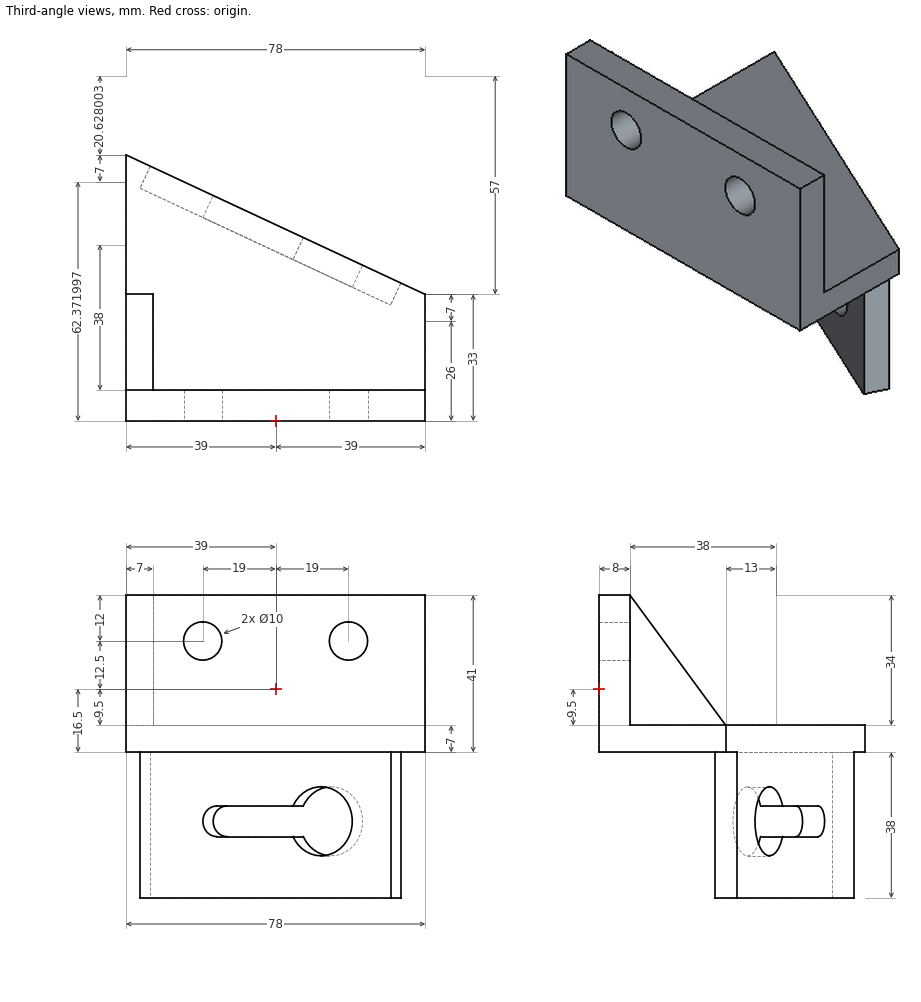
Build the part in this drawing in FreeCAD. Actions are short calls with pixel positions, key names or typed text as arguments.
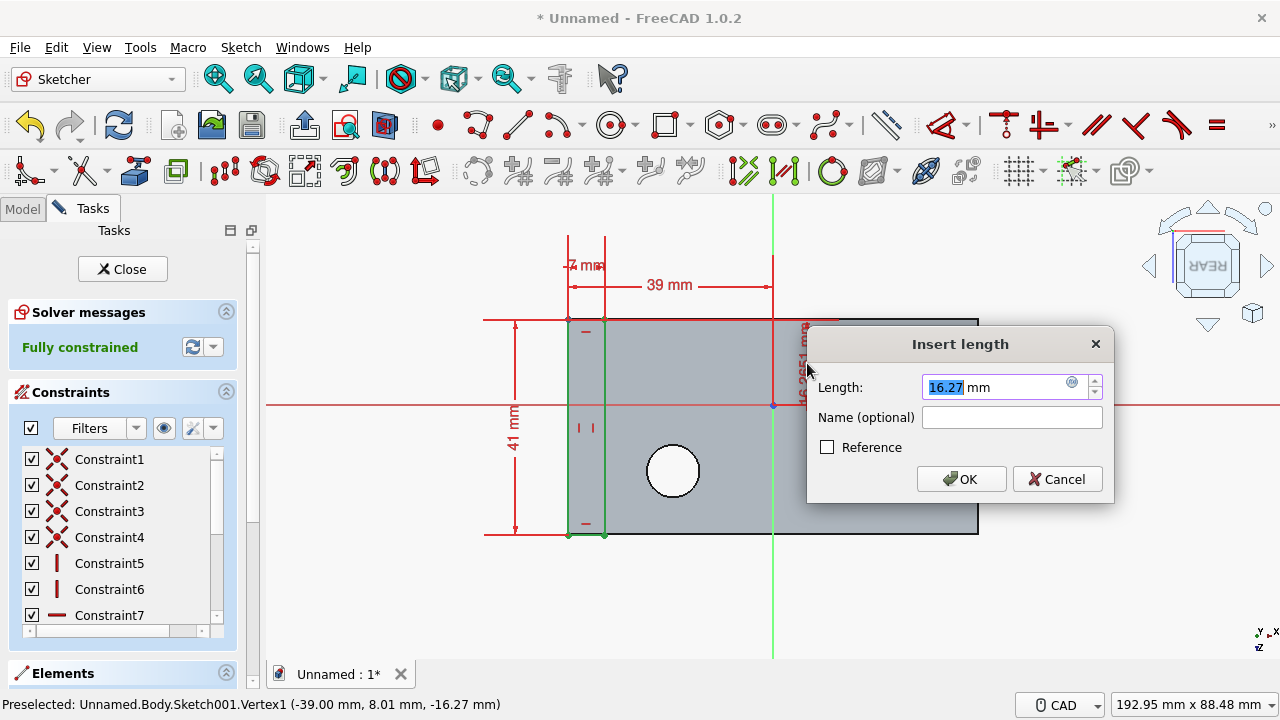
text(16.5)
key(Return)
key(Escape)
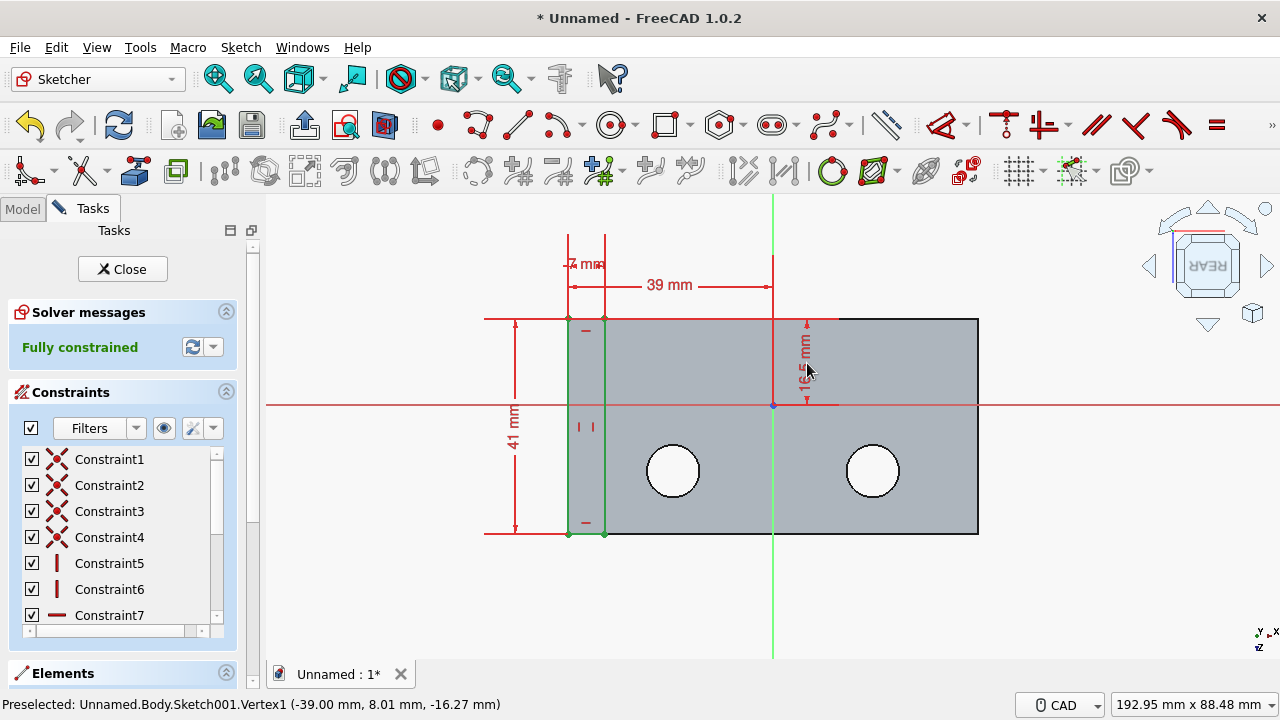
click(123, 269)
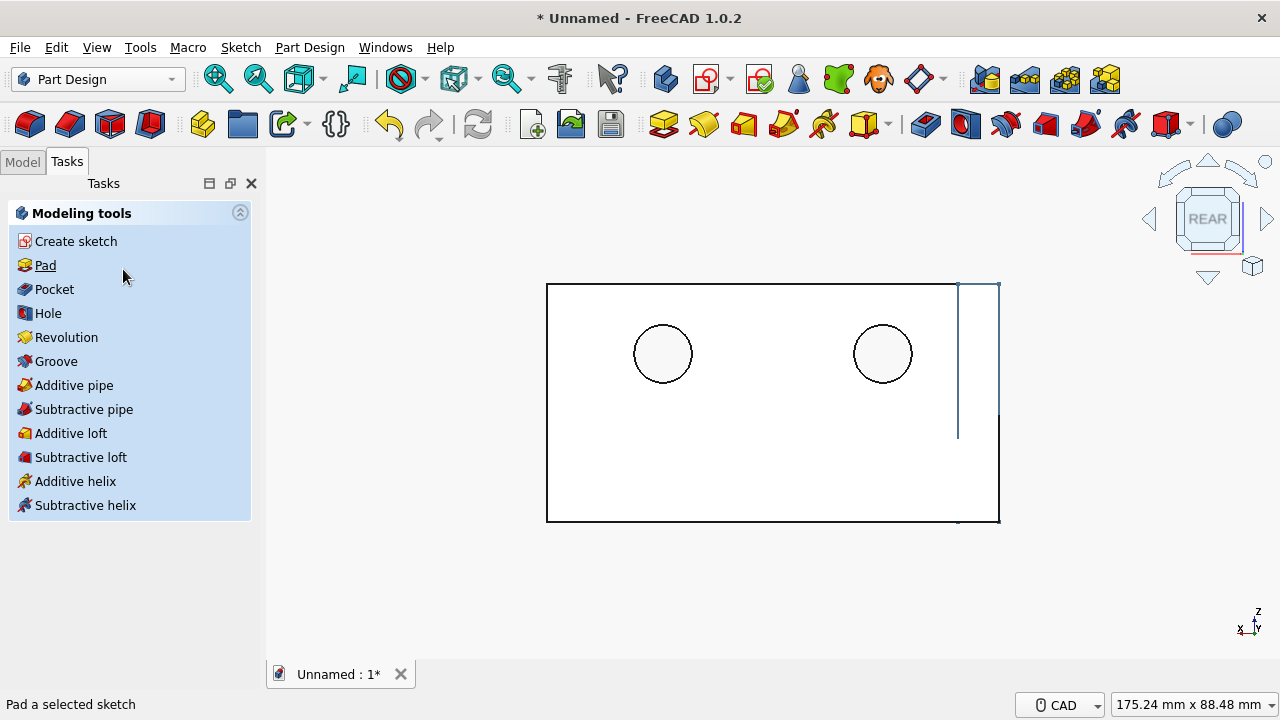
click(664, 124)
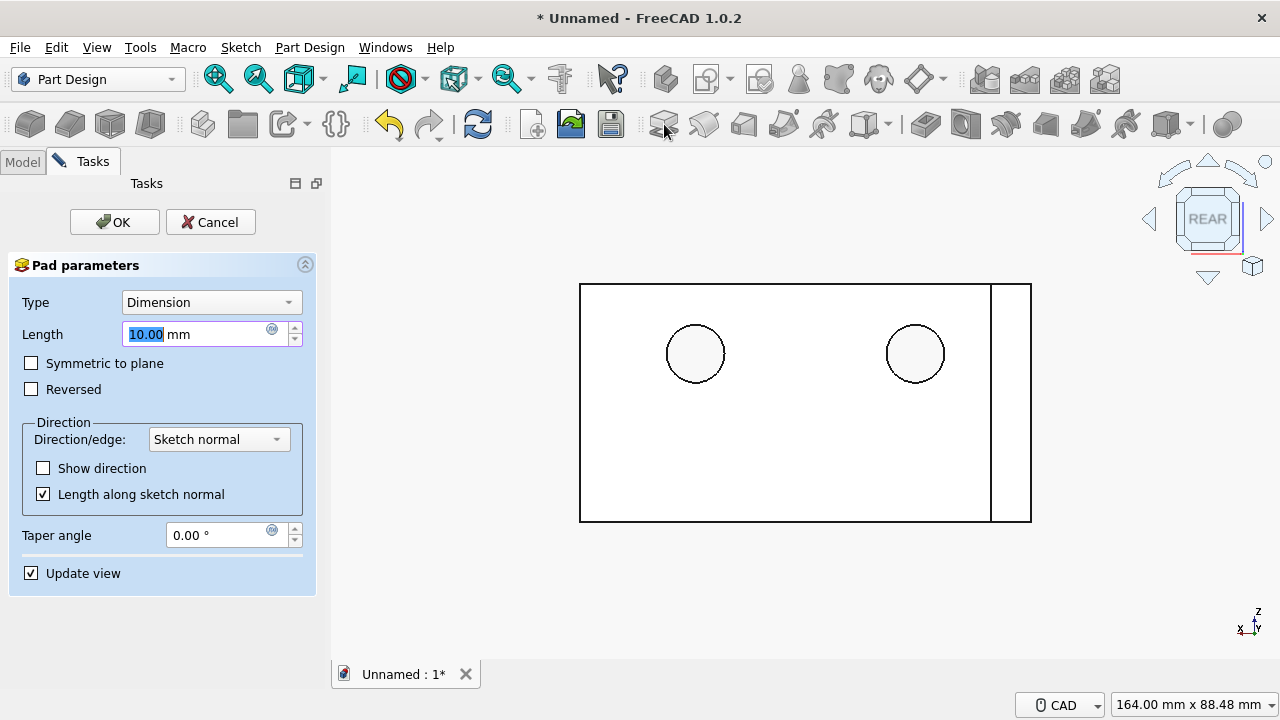
text(38)
key(Tab)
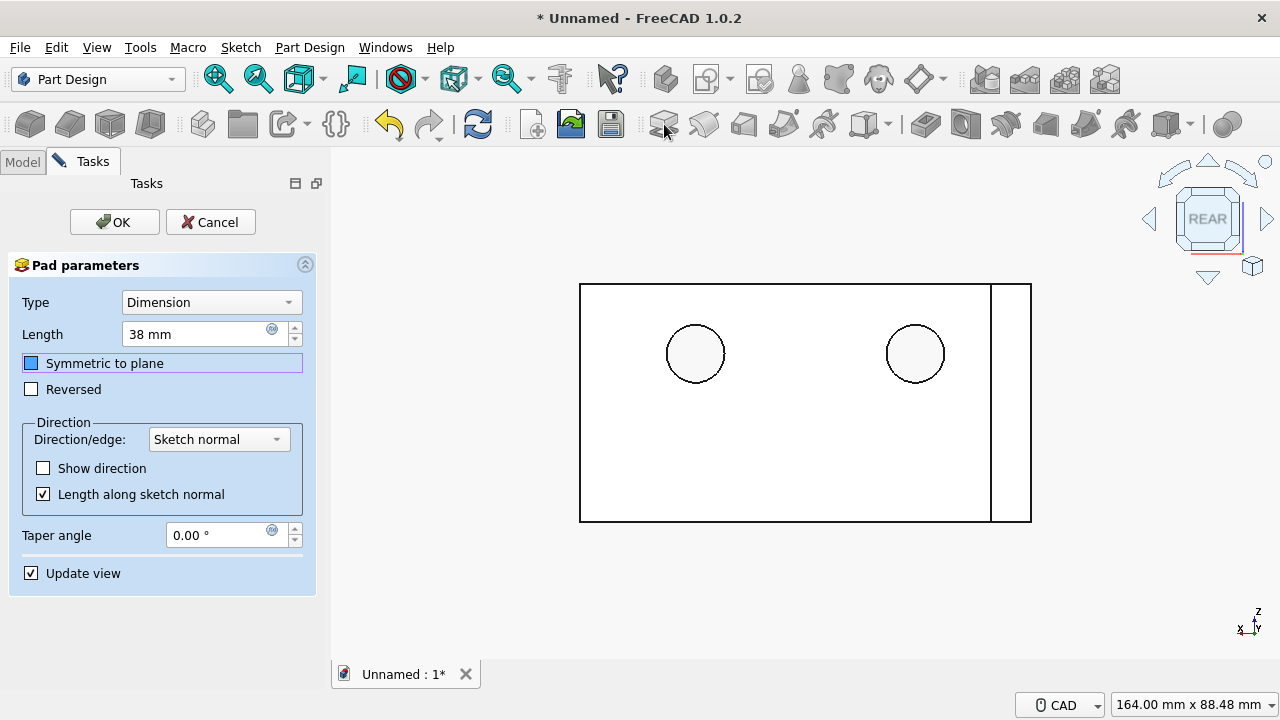
click(115, 222)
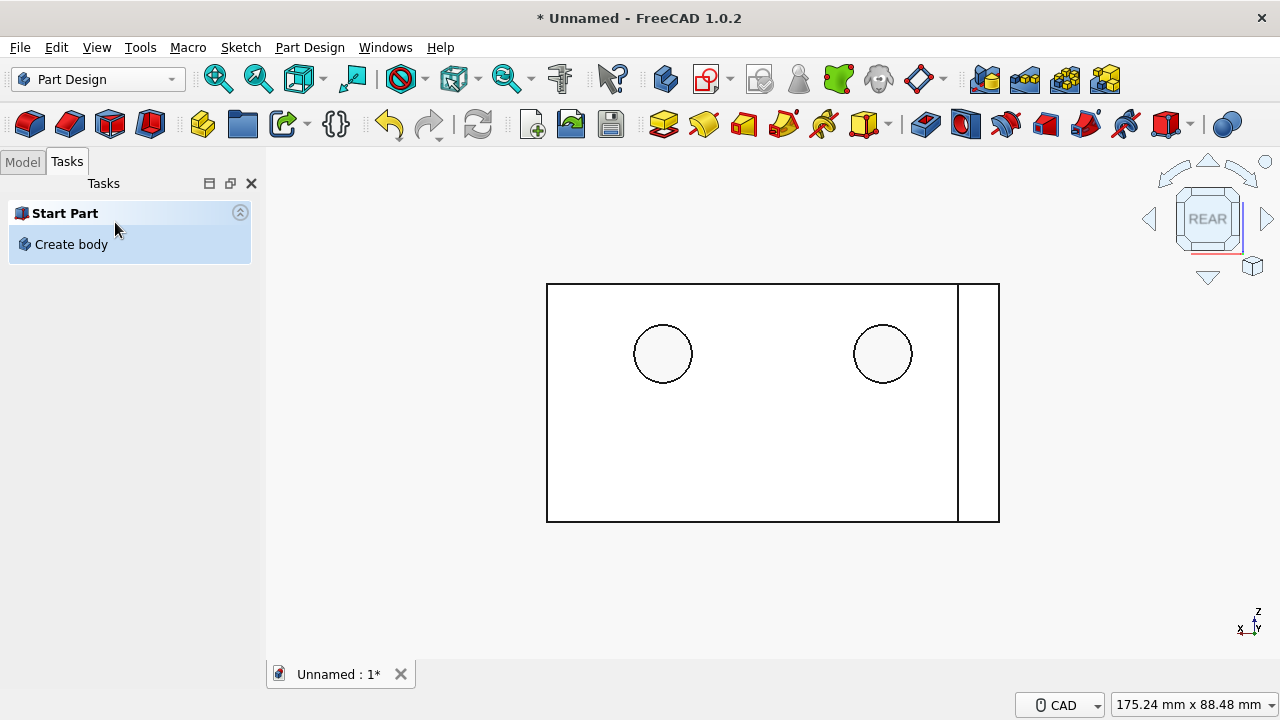
click(753, 436)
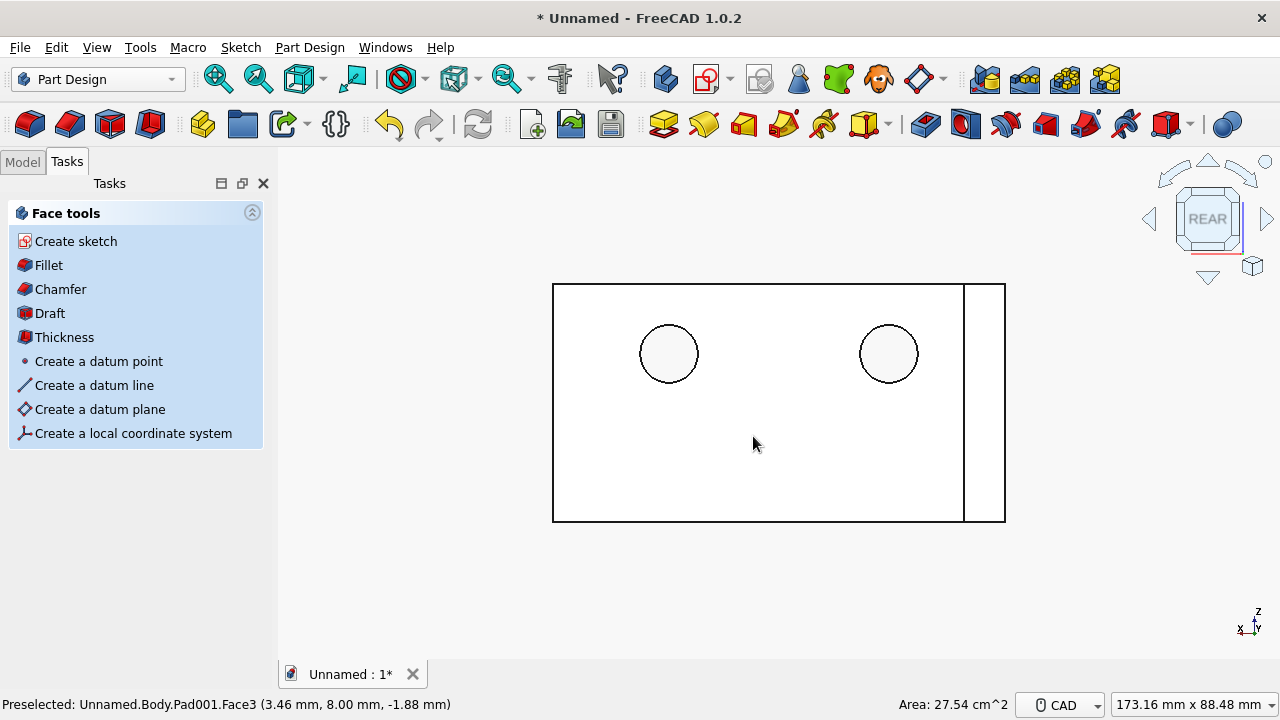
click(706, 80)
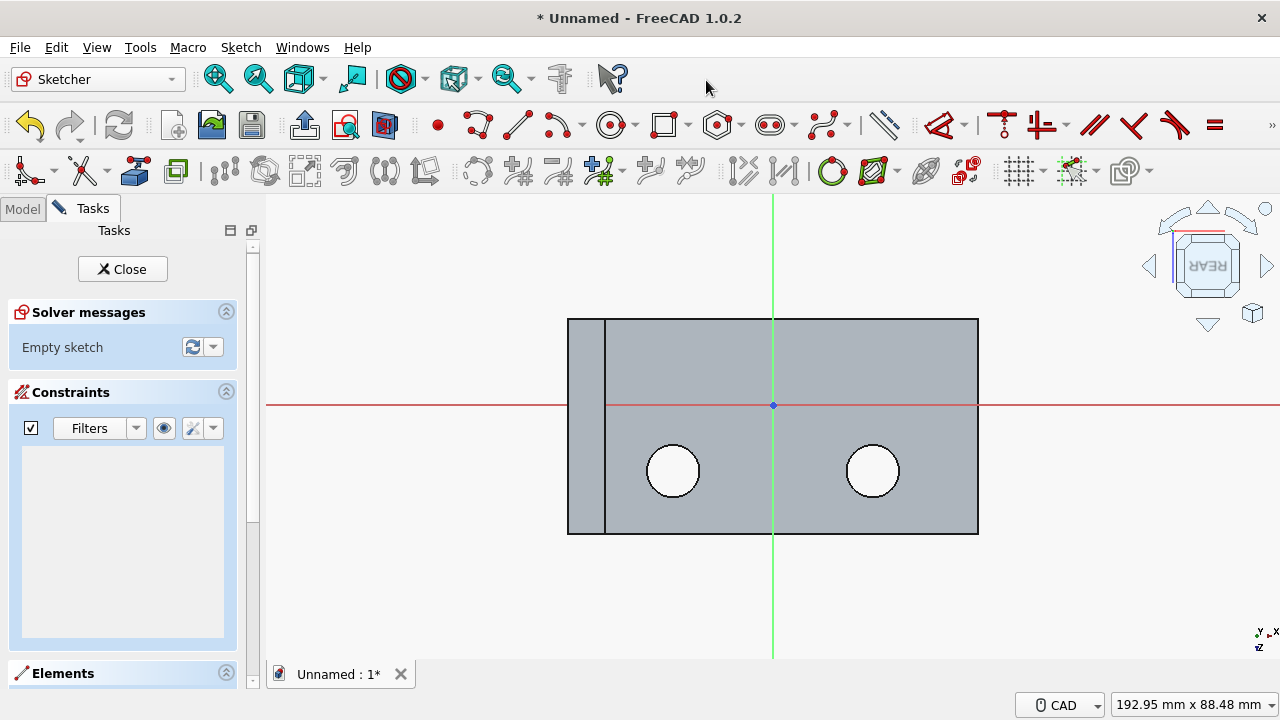
click(386, 126)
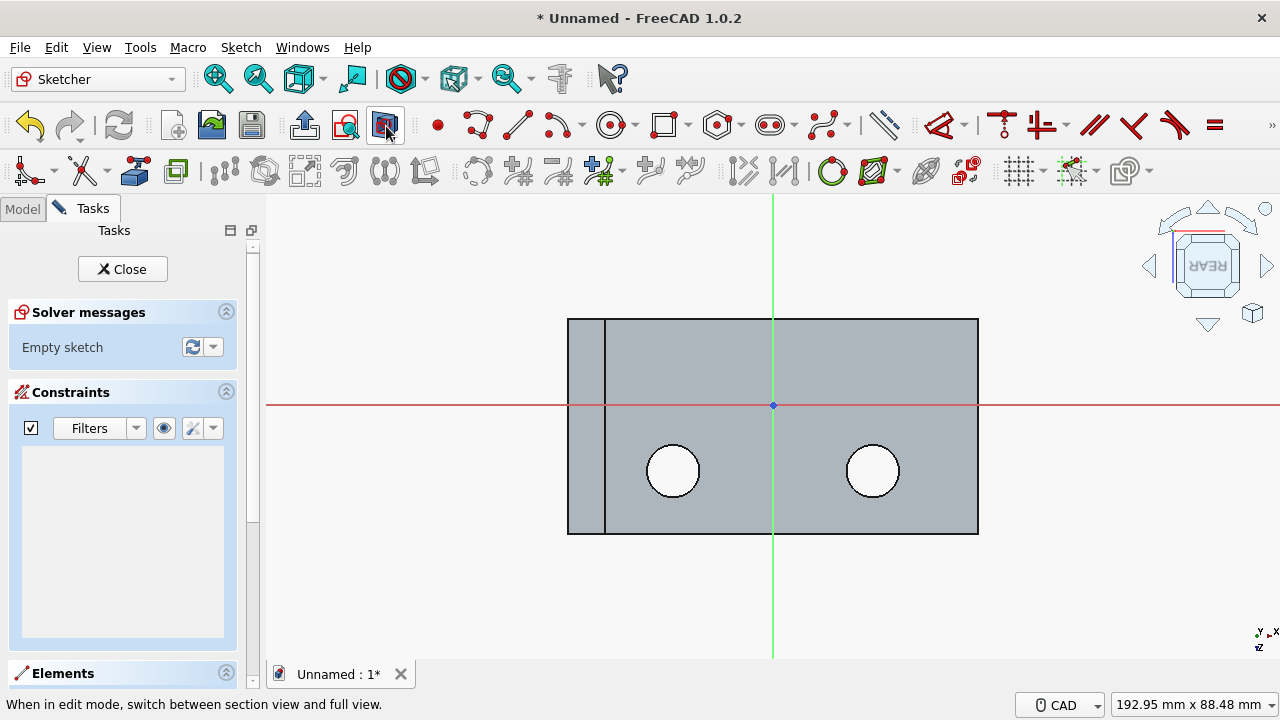
scroll(912, 231, up, 2)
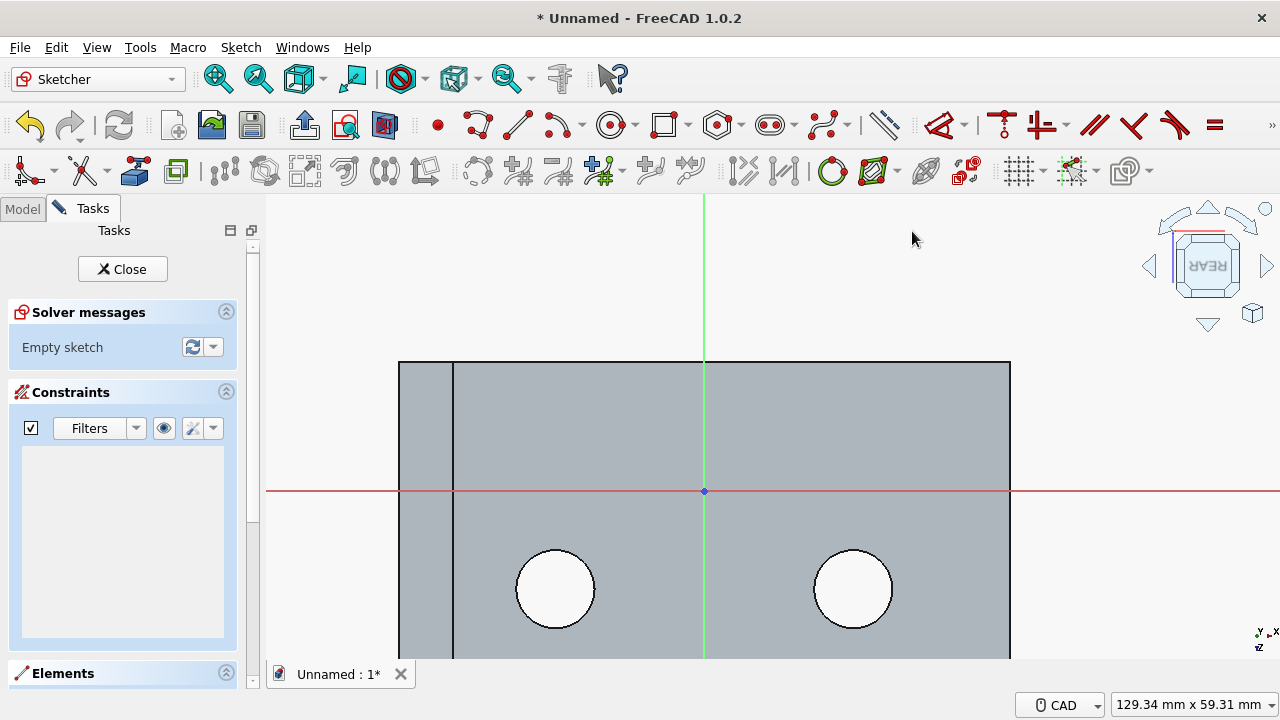
click(664, 126)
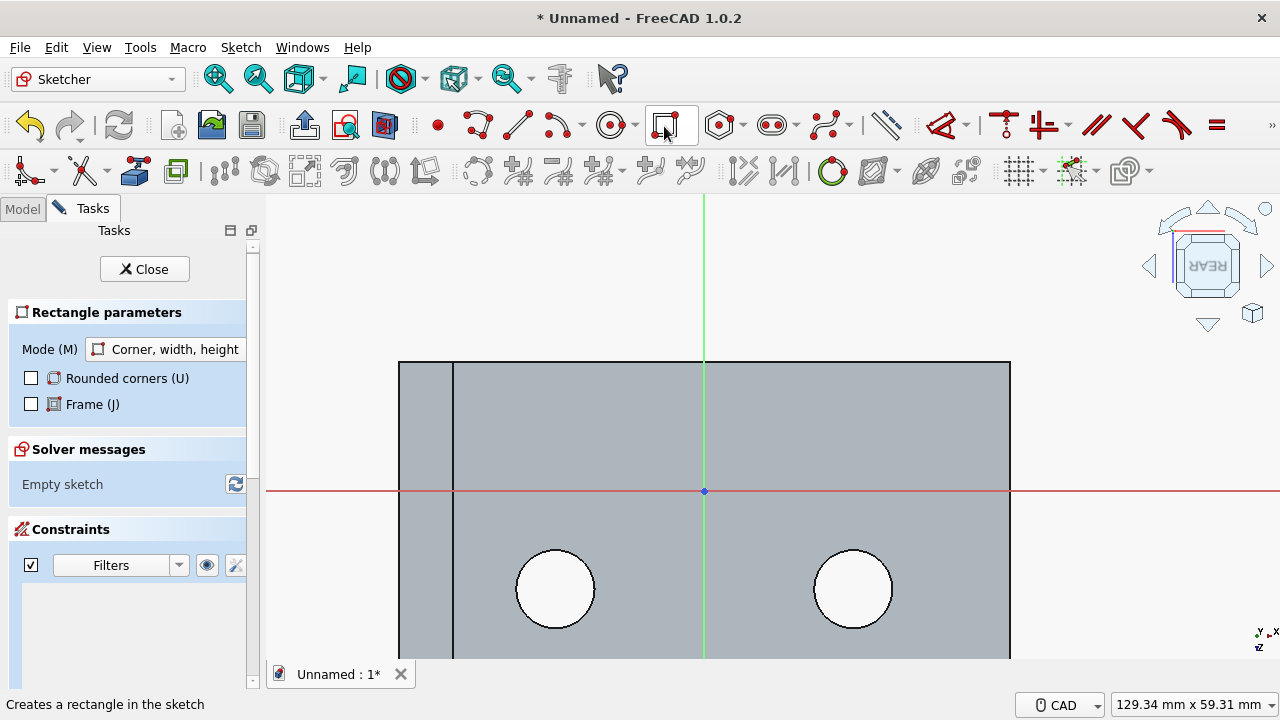
click(399, 362)
move(1010, 417)